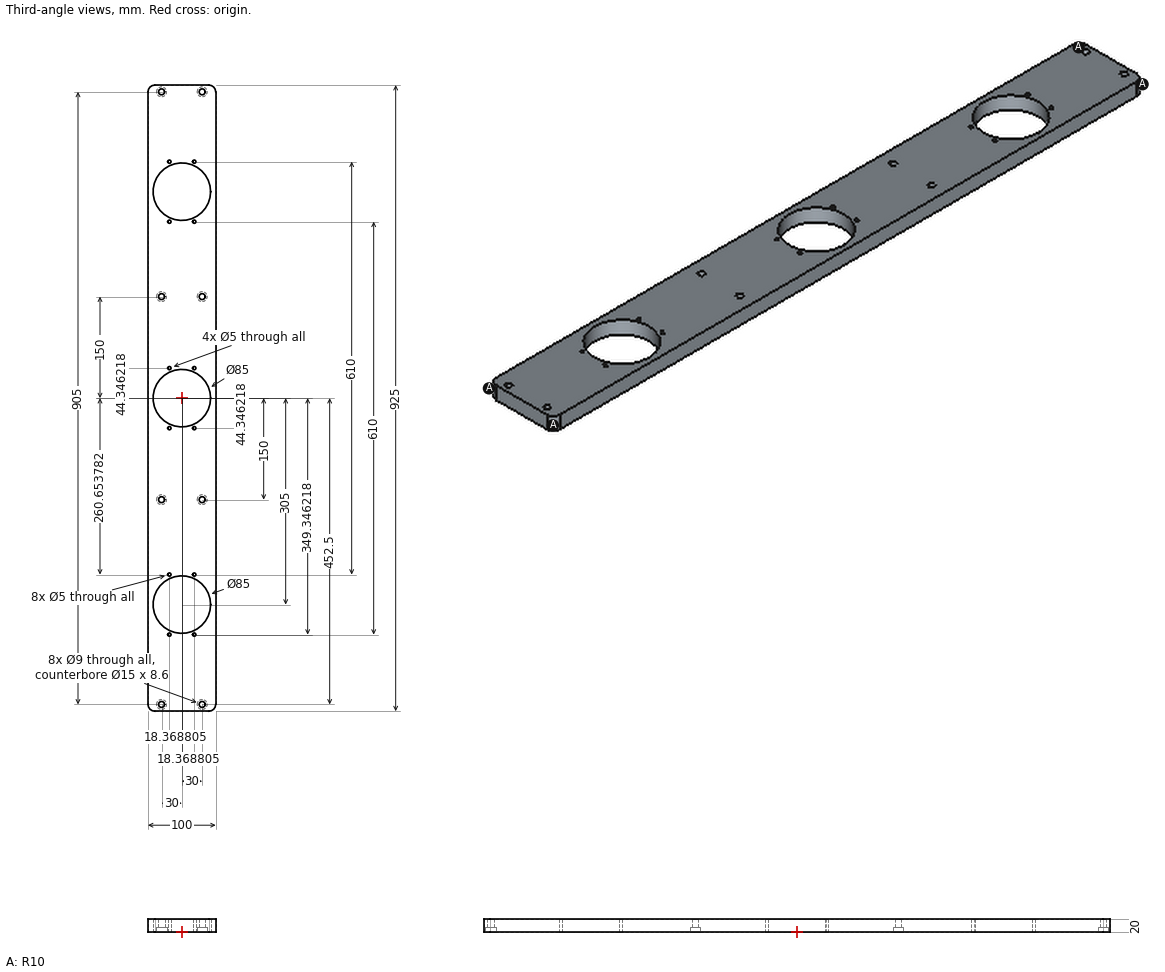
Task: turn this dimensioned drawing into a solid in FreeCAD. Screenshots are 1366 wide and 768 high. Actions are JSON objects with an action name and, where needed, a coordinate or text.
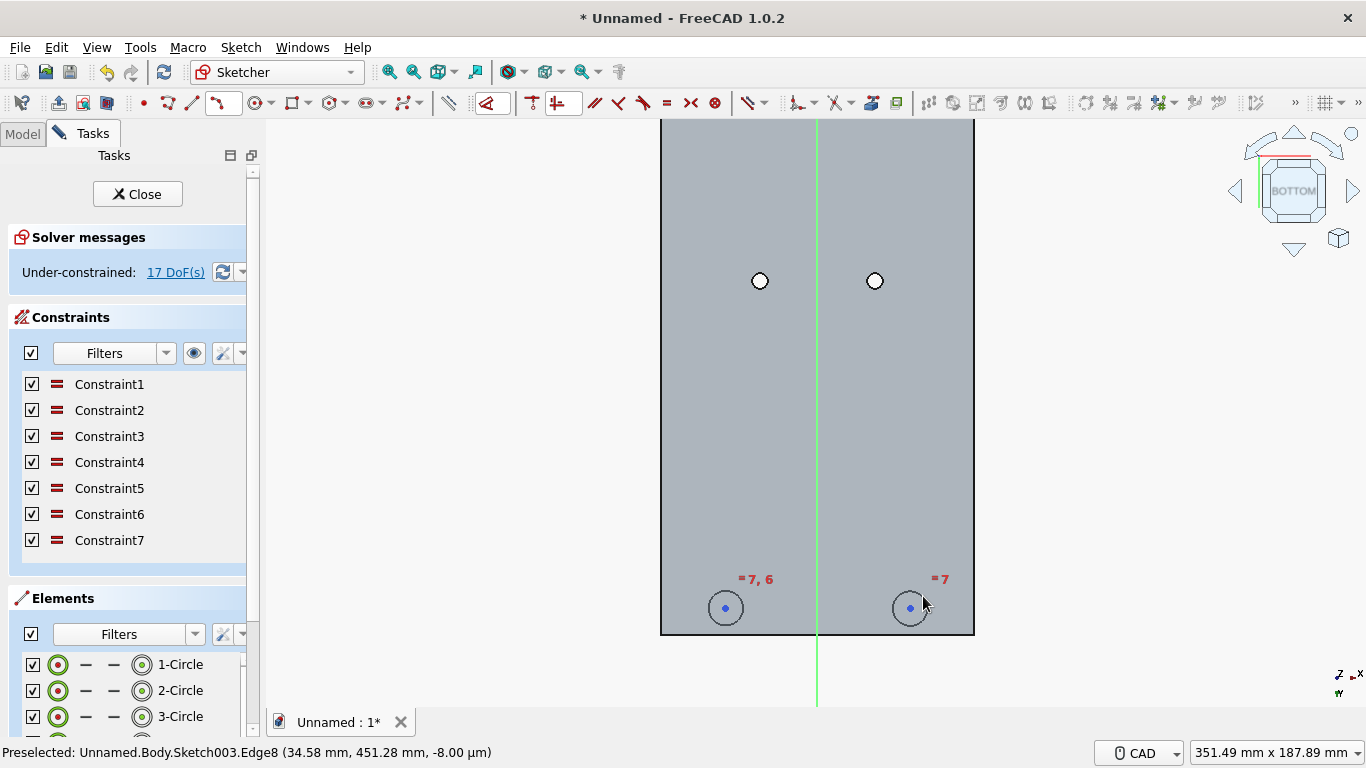
{"action": "key", "text": "d"}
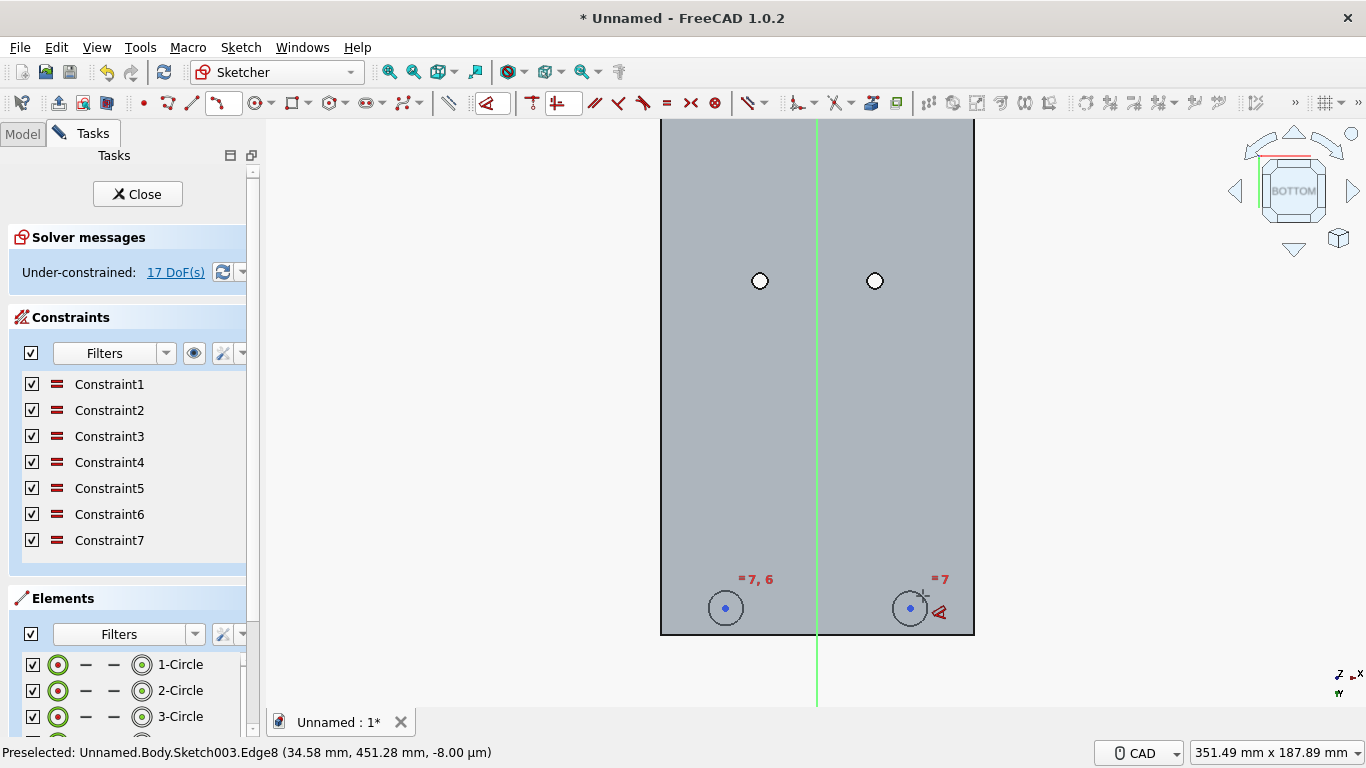
{"action": "scroll", "coordinate": [737, 605], "scroll_direction": "down", "scroll_amount": 10}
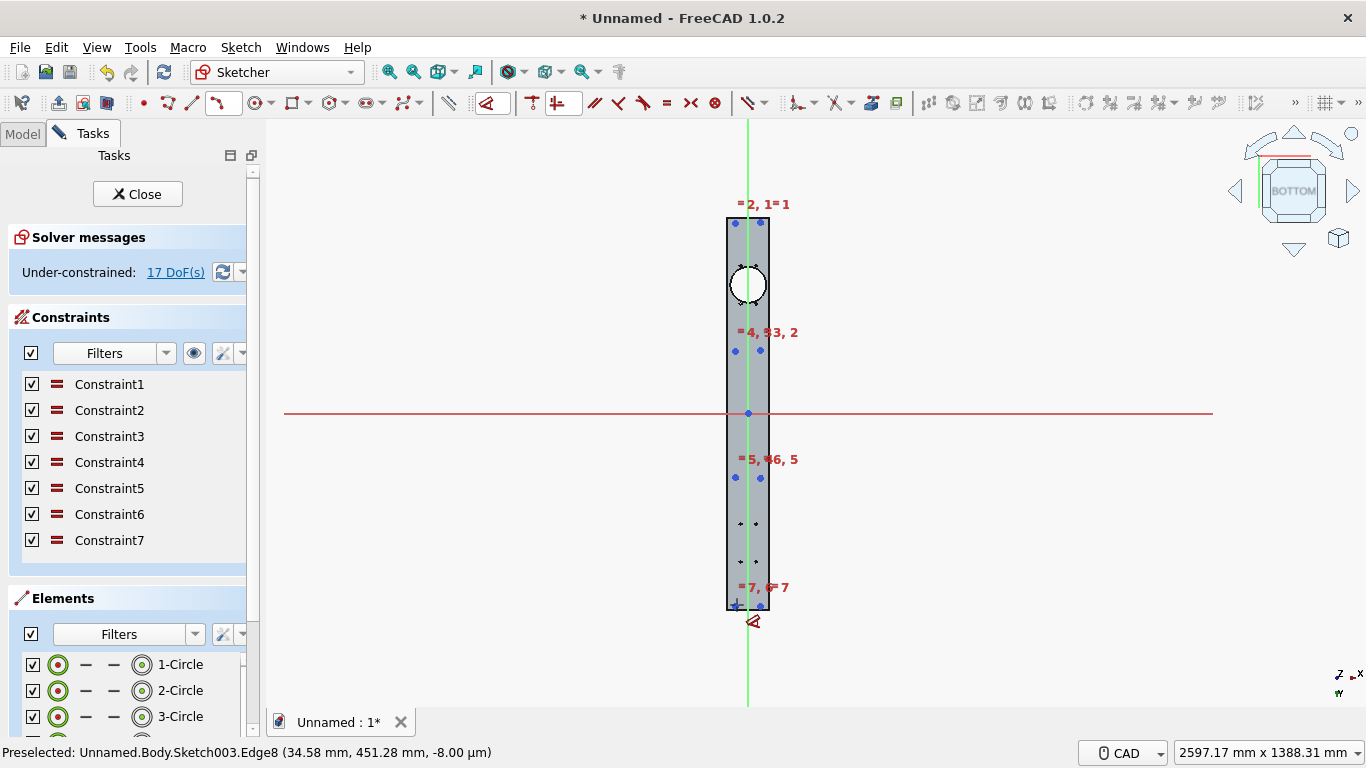
{"action": "scroll", "coordinate": [763, 221], "scroll_direction": "up", "scroll_amount": 12}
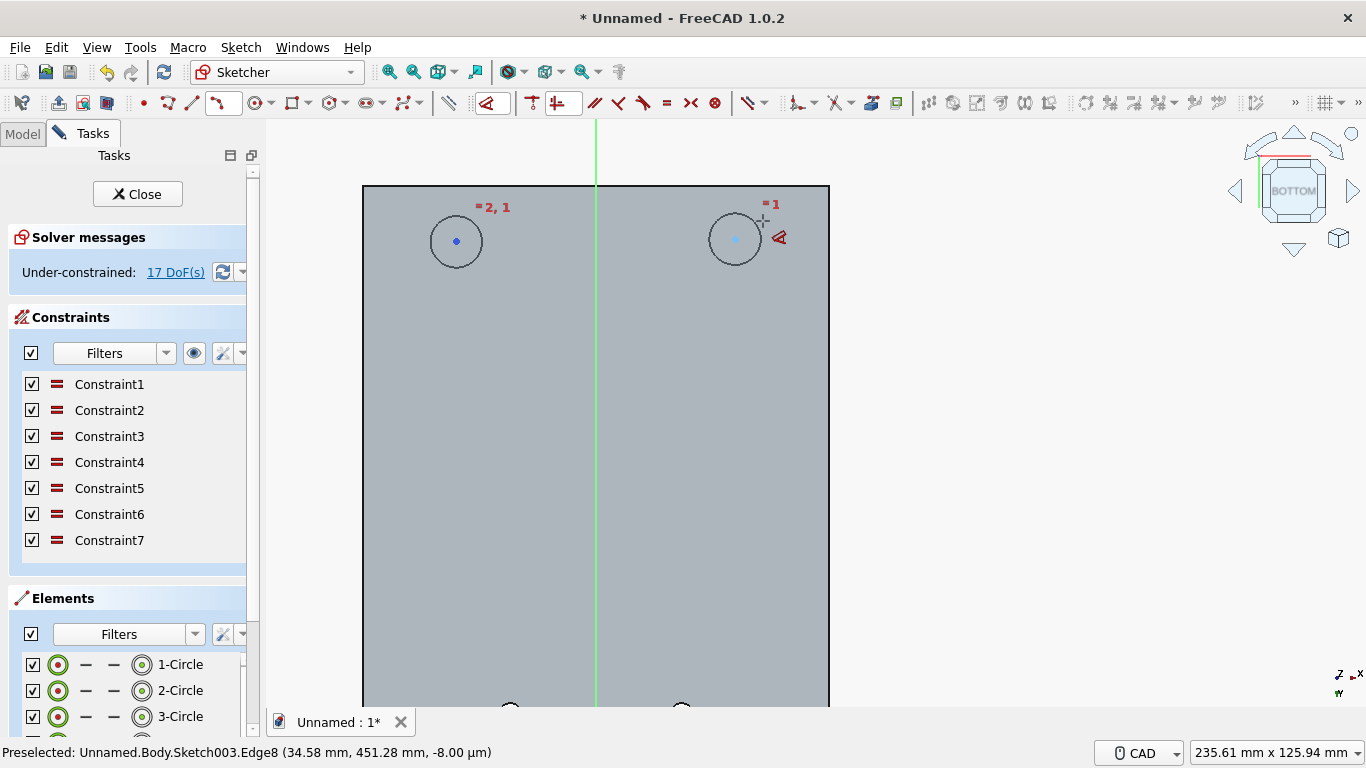
{"action": "left_click", "coordinate": [753, 221]}
{"action": "left_click", "coordinate": [775, 198]}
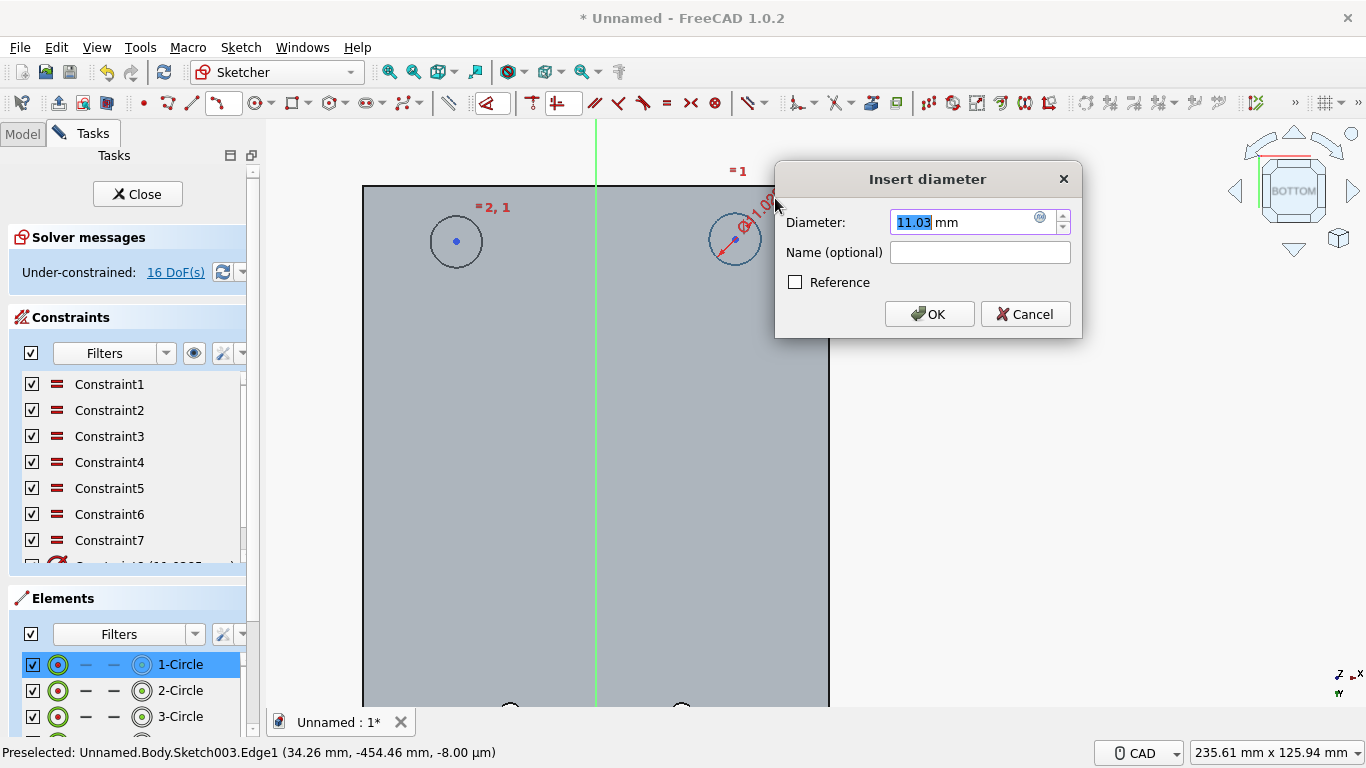
{"action": "type", "text": "9"}
{"action": "key", "text": "Return"}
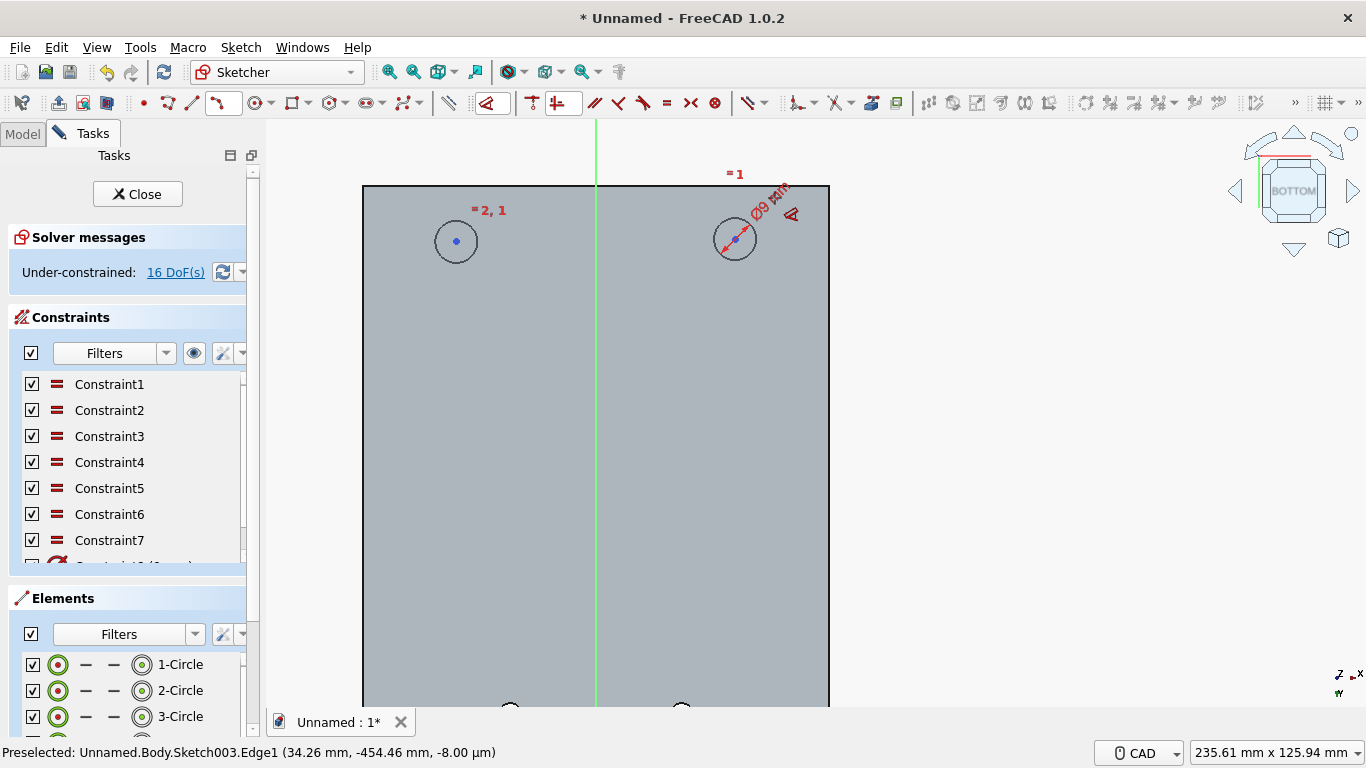
{"action": "scroll", "coordinate": [763, 220], "scroll_direction": "down", "scroll_amount": 12}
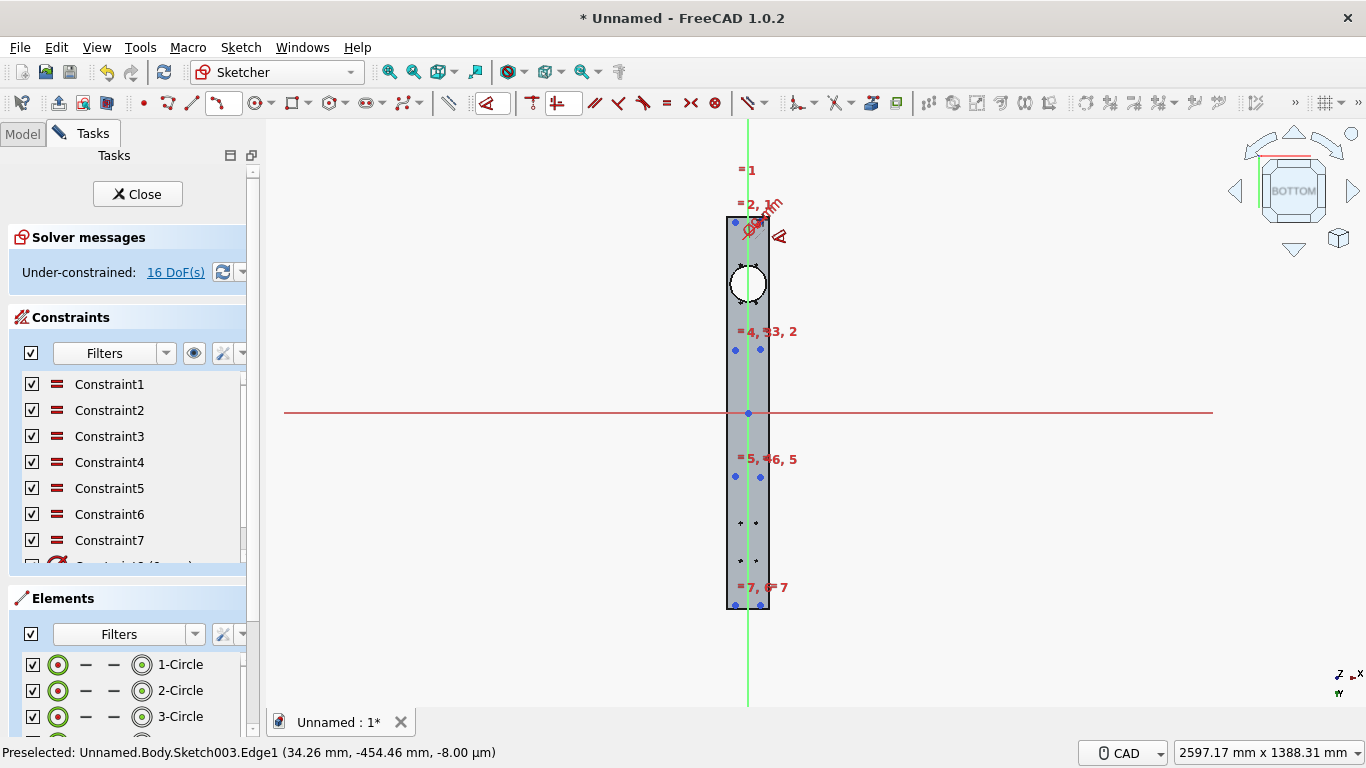
{"action": "scroll", "coordinate": [761, 222], "scroll_direction": "up", "scroll_amount": 6}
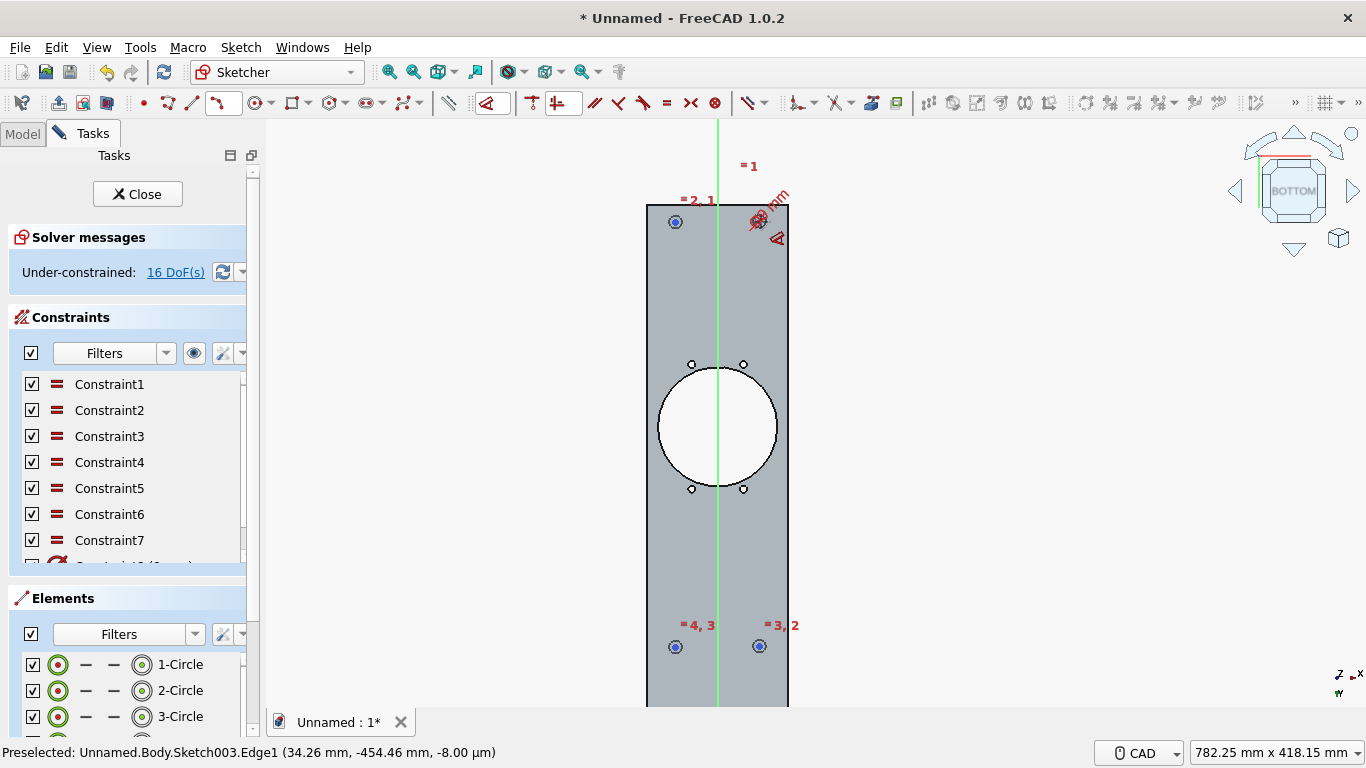
{"action": "left_click", "coordinate": [760, 221]}
{"action": "left_click", "coordinate": [739, 187]}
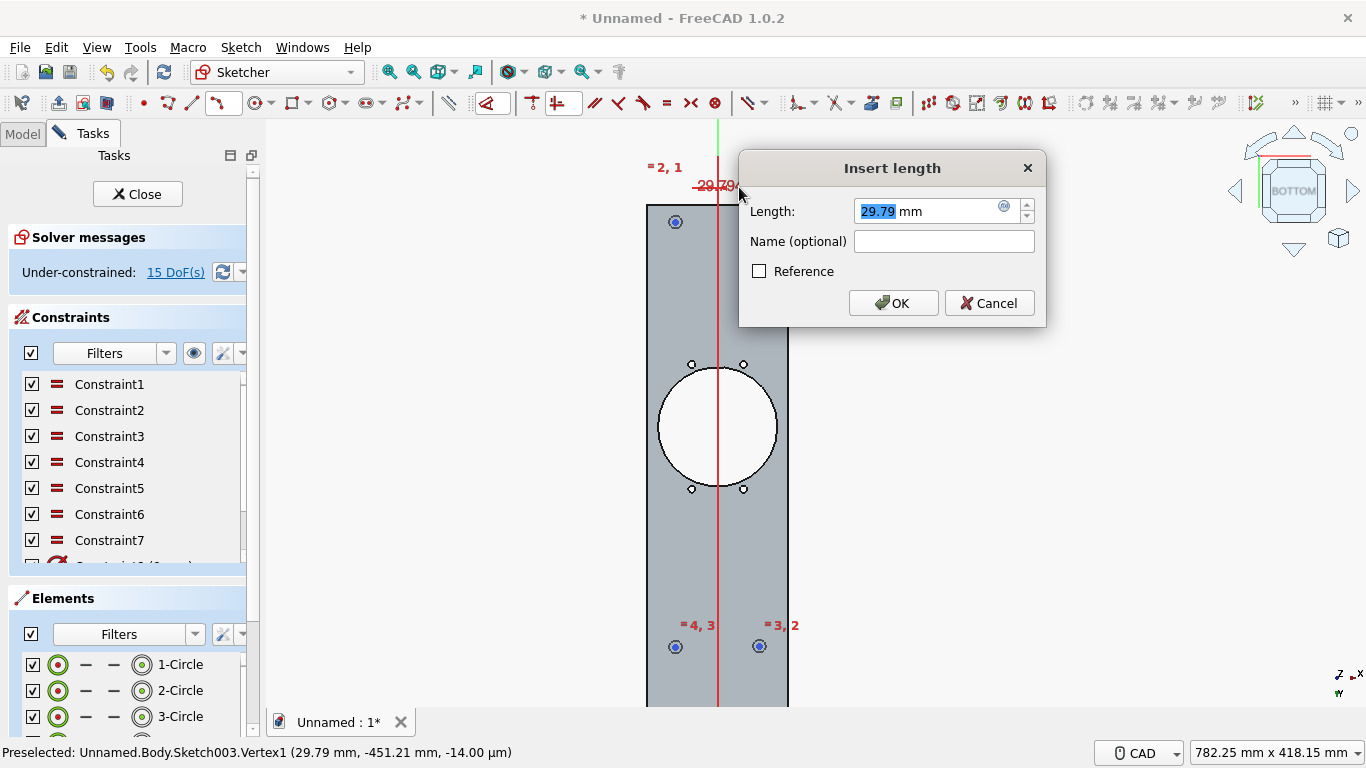
{"action": "type", "text": "30"}
{"action": "key", "text": "Return"}